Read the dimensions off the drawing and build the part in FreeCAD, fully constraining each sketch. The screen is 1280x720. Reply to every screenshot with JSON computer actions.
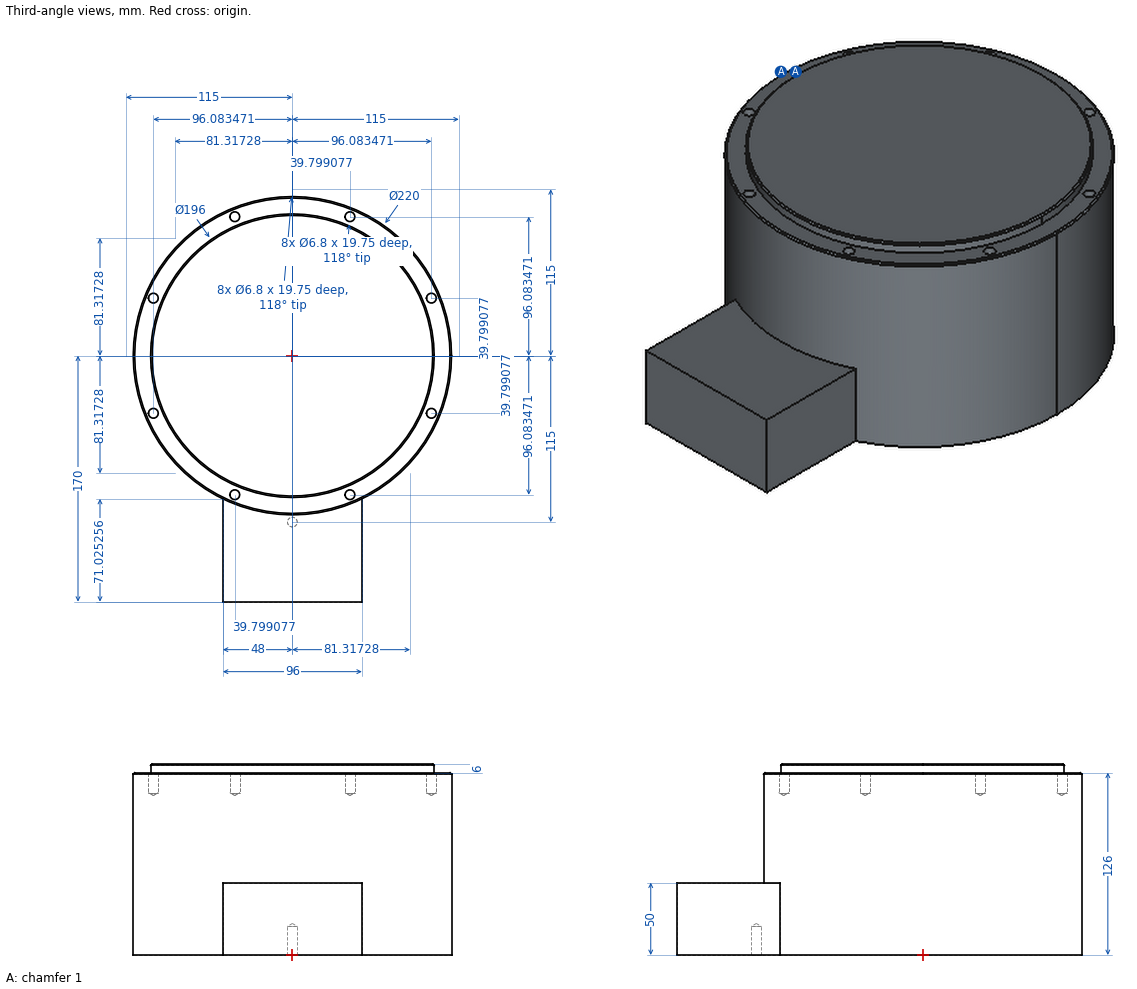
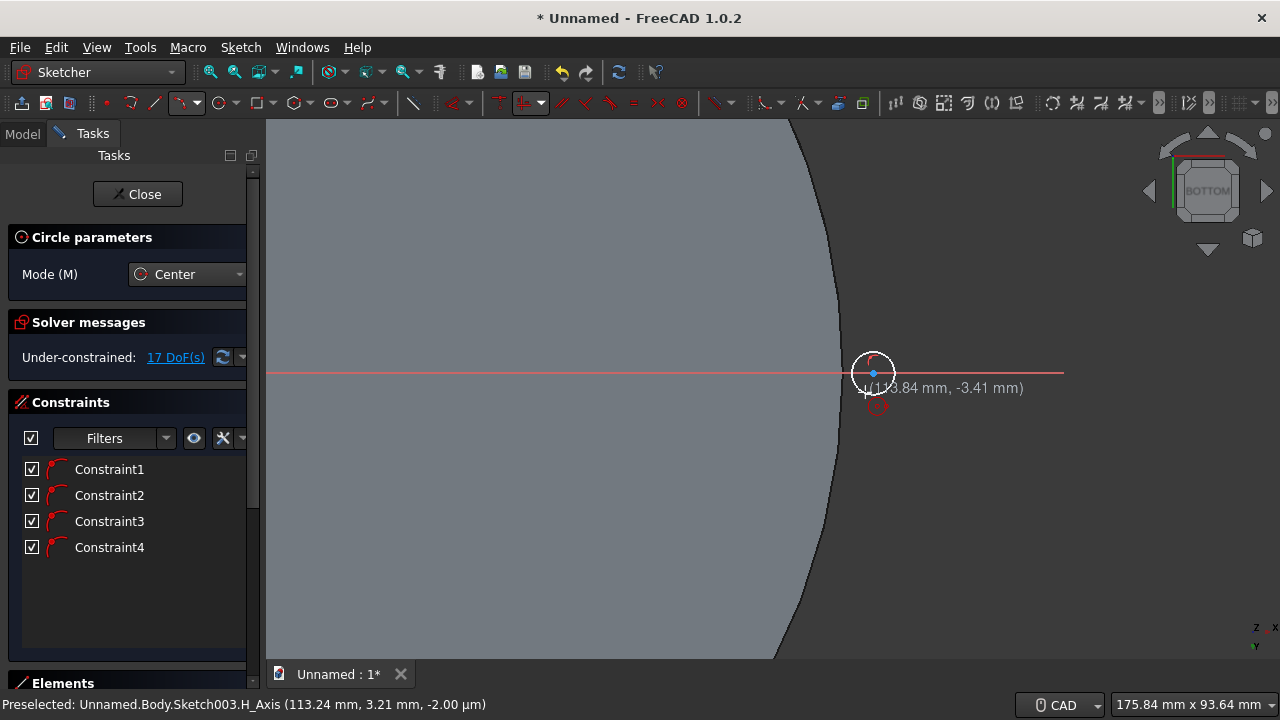
{"action": "scroll", "coordinate": [867, 394], "scroll_direction": "down", "scroll_amount": 7}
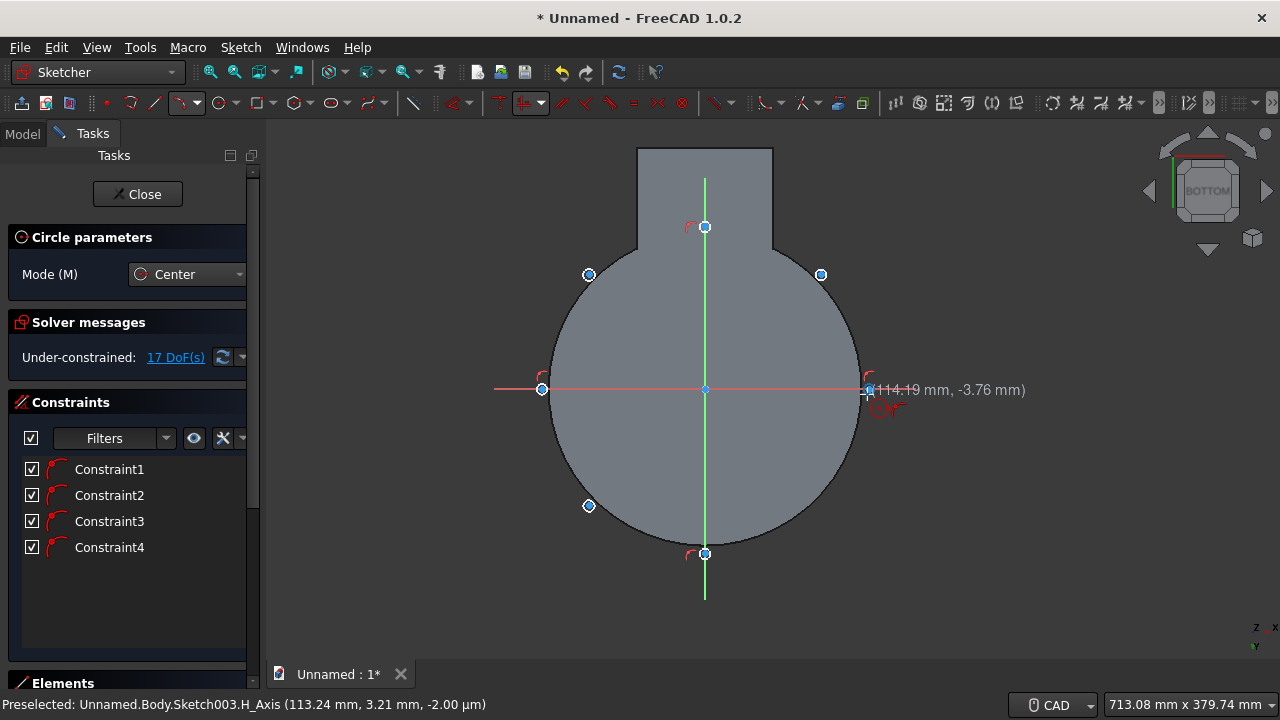
{"action": "scroll", "coordinate": [821, 505], "scroll_direction": "up", "scroll_amount": 8}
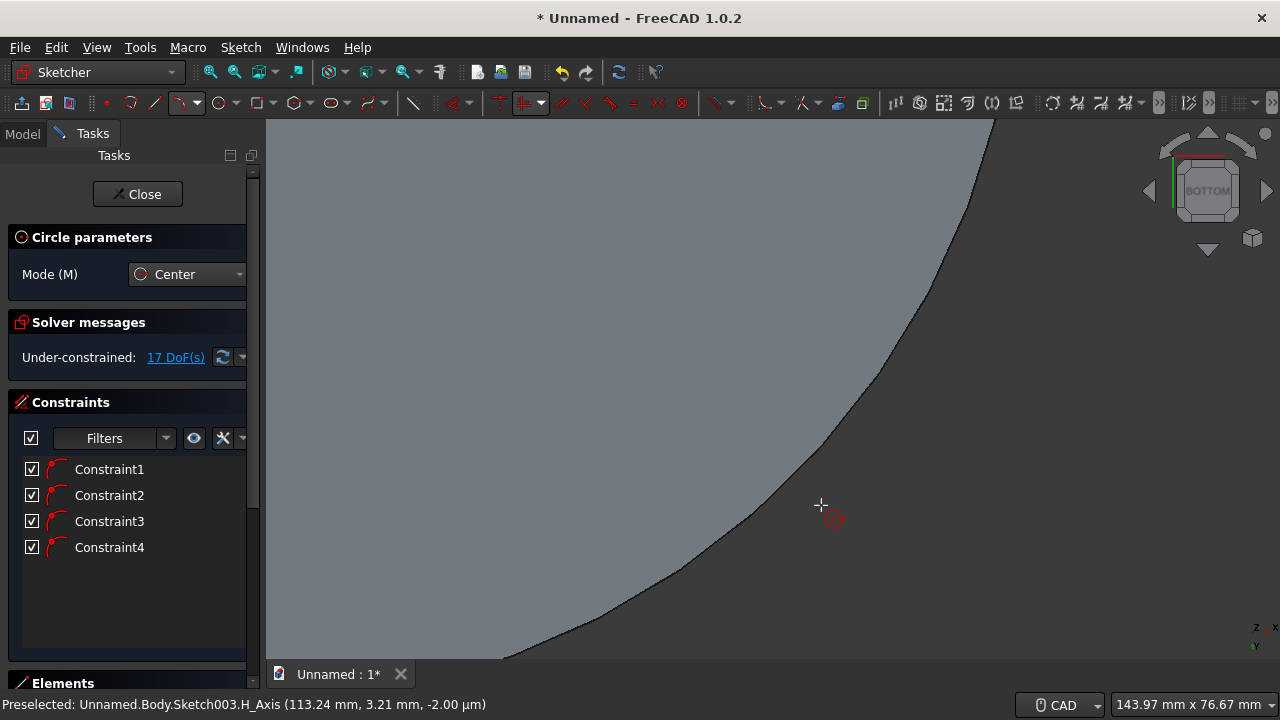
{"action": "scroll", "coordinate": [821, 505], "scroll_direction": "down", "scroll_amount": 8}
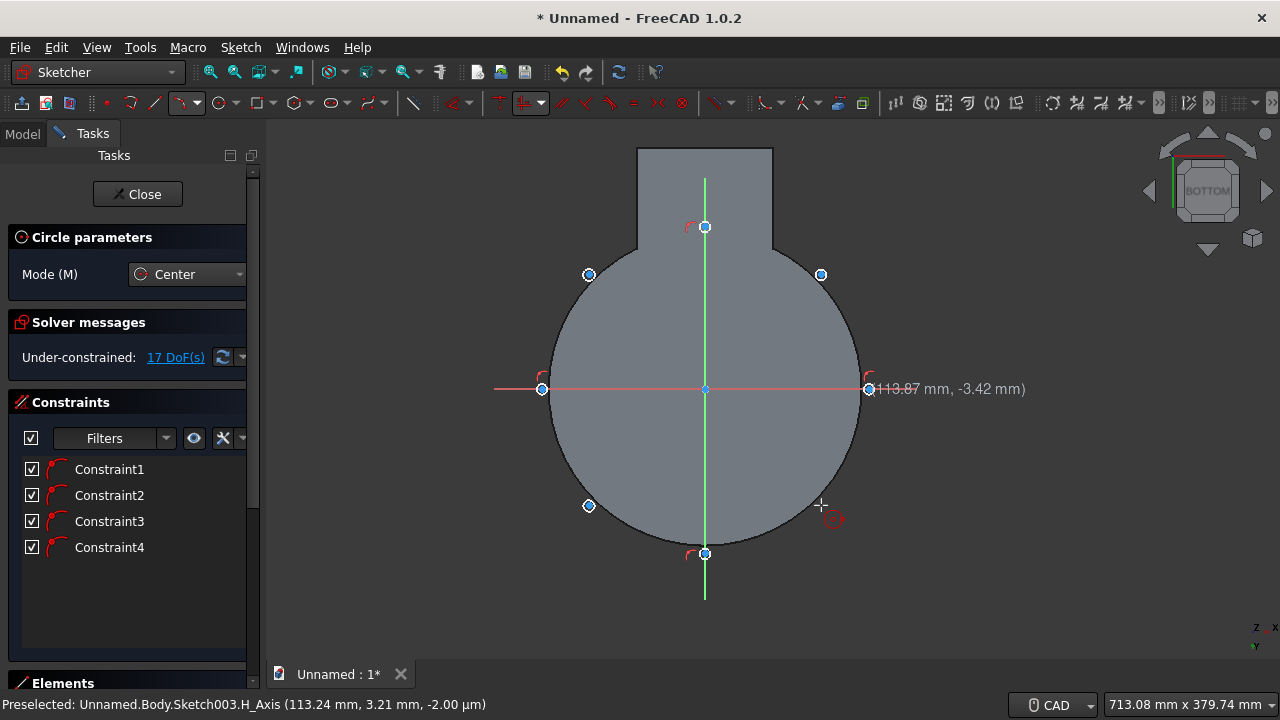
{"action": "left_click", "coordinate": [821, 505]}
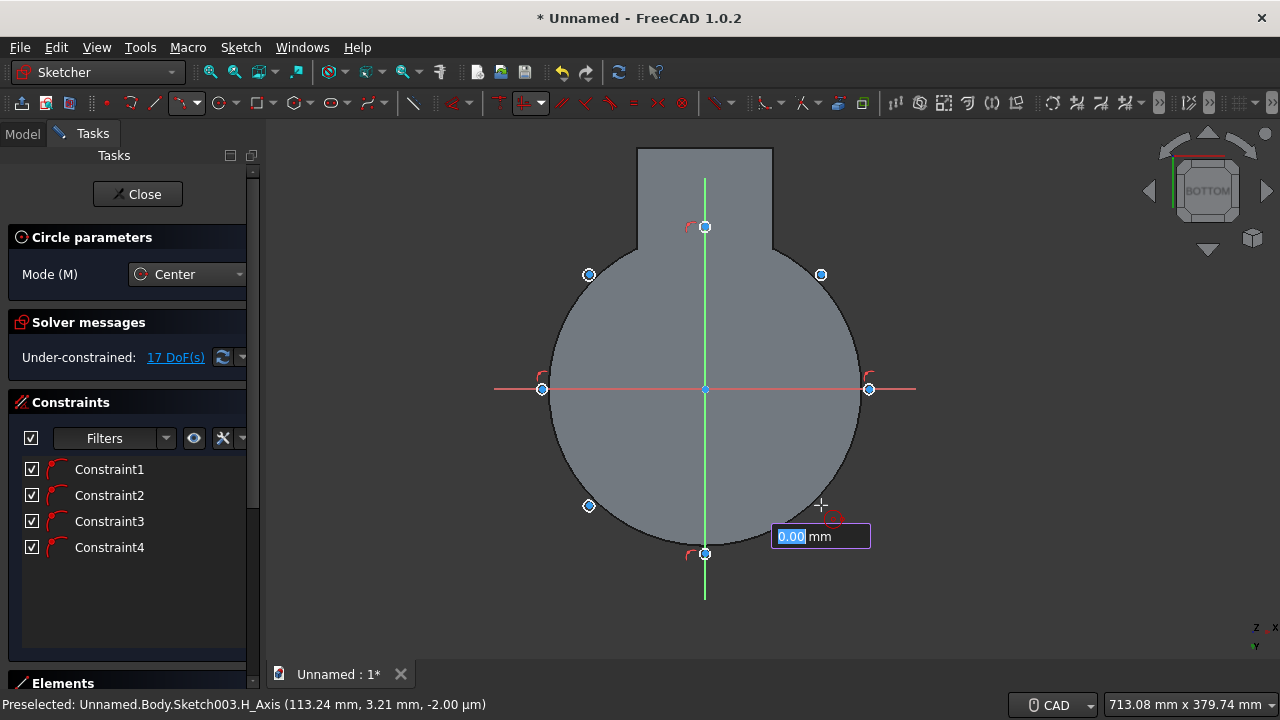
{"action": "scroll", "coordinate": [824, 502], "scroll_direction": "up", "scroll_amount": 6}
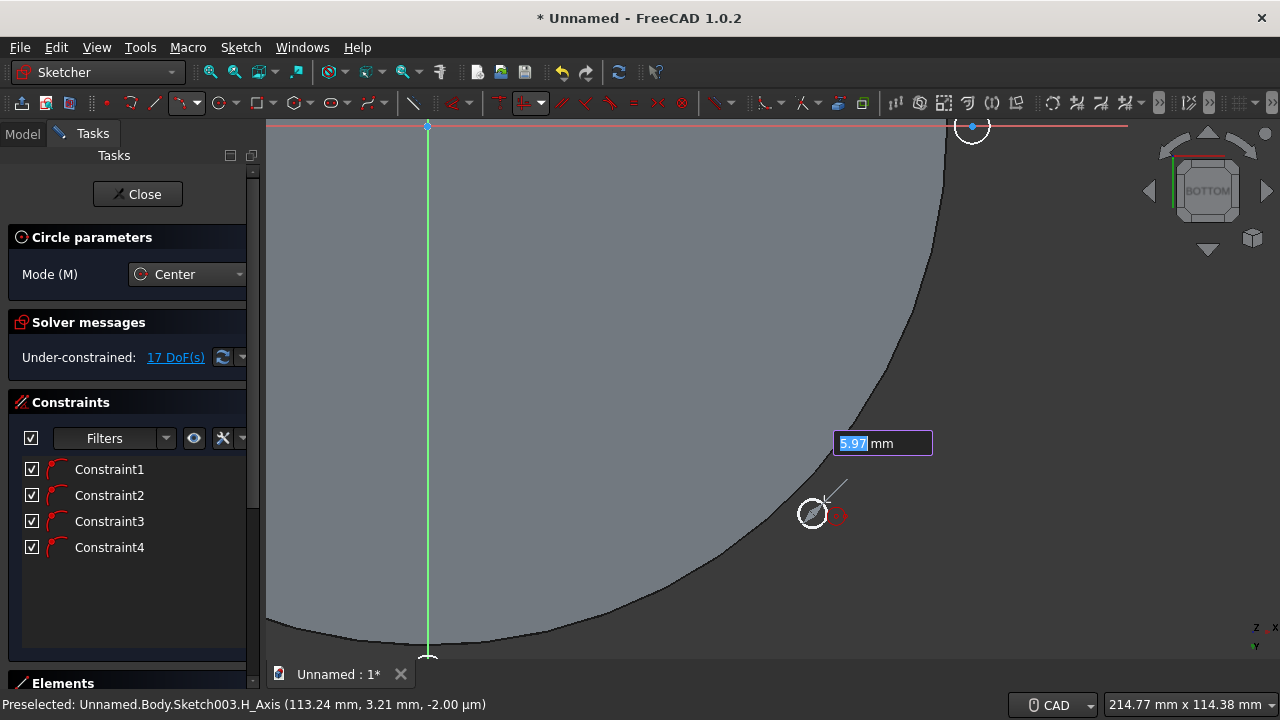
{"action": "left_click", "coordinate": [823, 499]}
{"action": "key", "text": "Escape"}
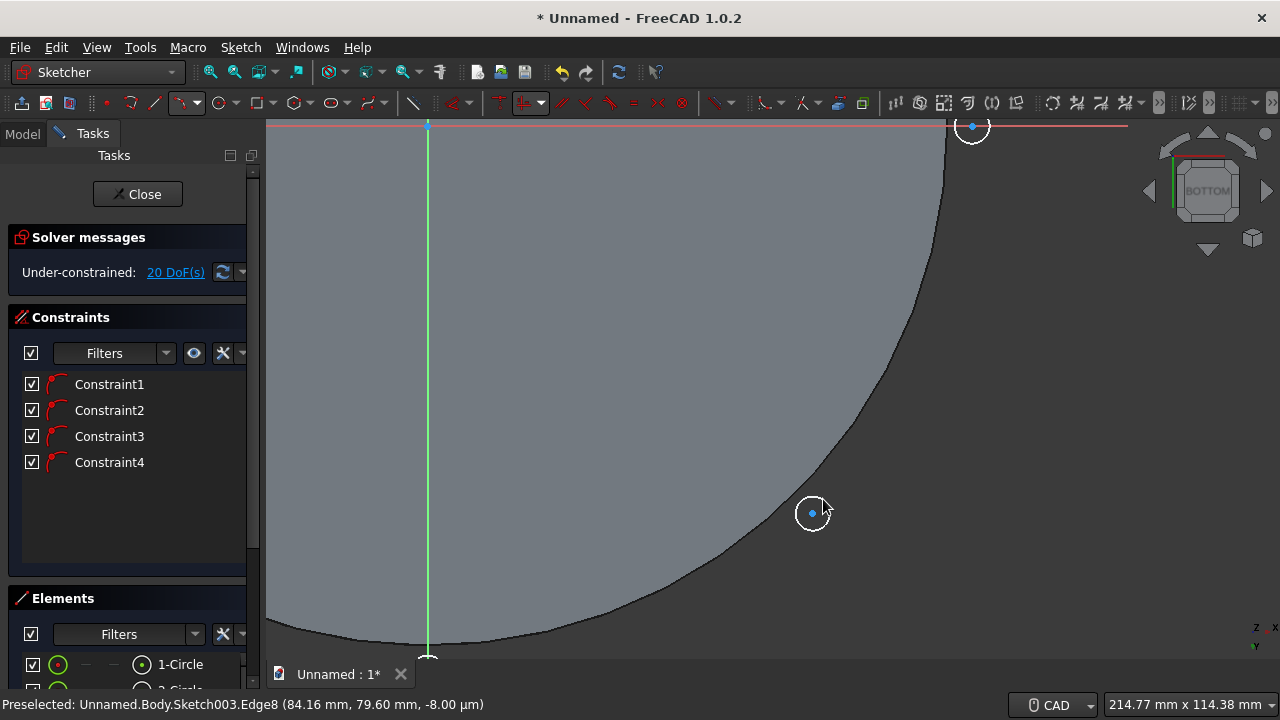
{"action": "scroll", "coordinate": [824, 502], "scroll_direction": "down", "scroll_amount": 6}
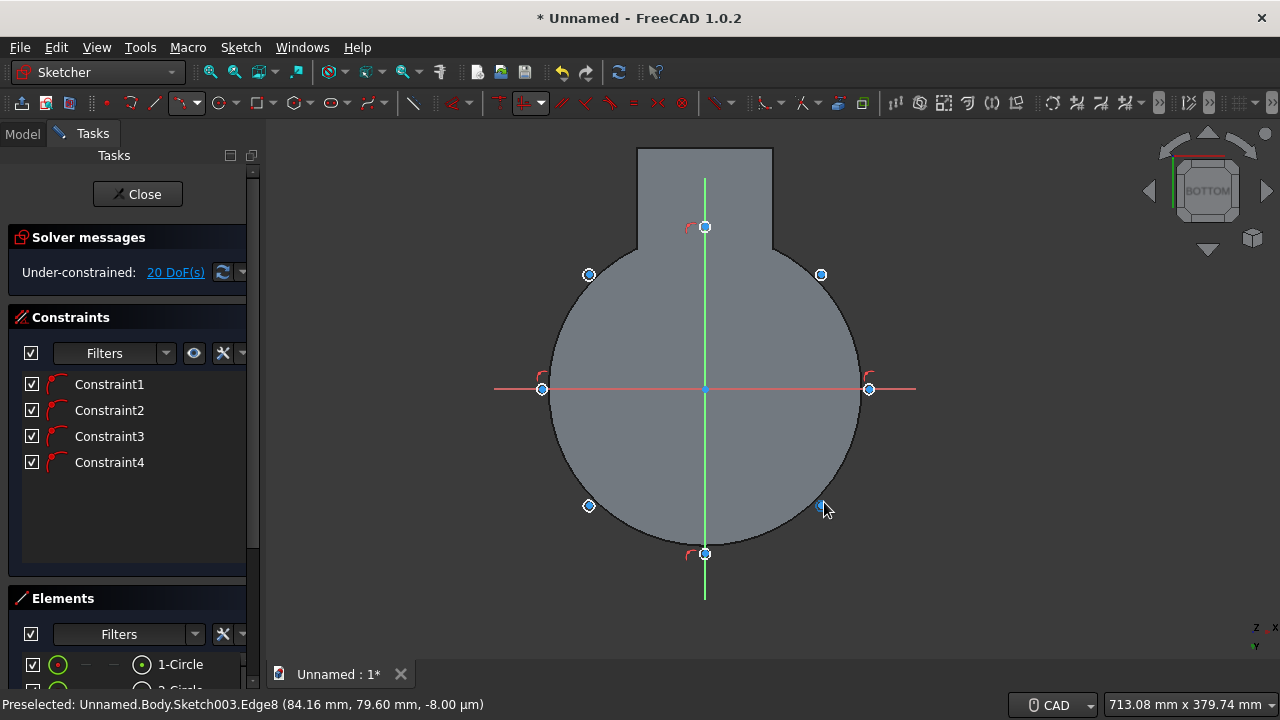
{"action": "scroll", "coordinate": [709, 550], "scroll_direction": "up", "scroll_amount": 7}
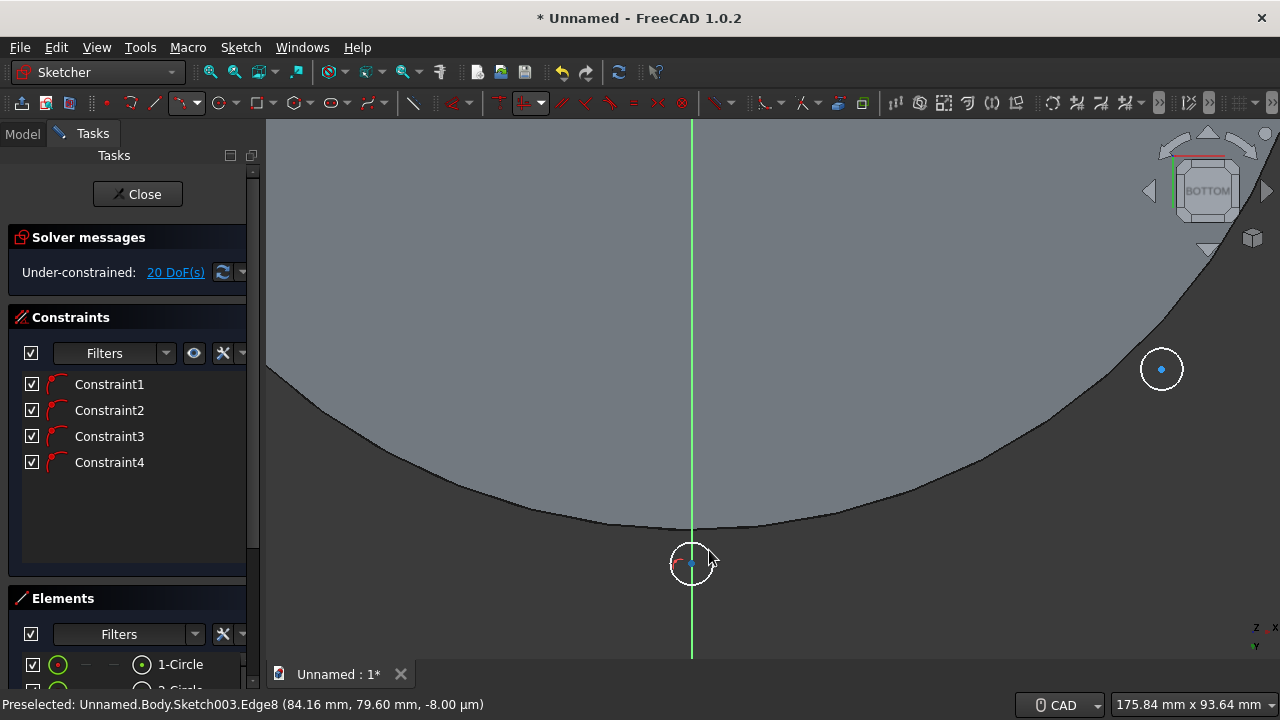
{"action": "left_click", "coordinate": [707, 549]}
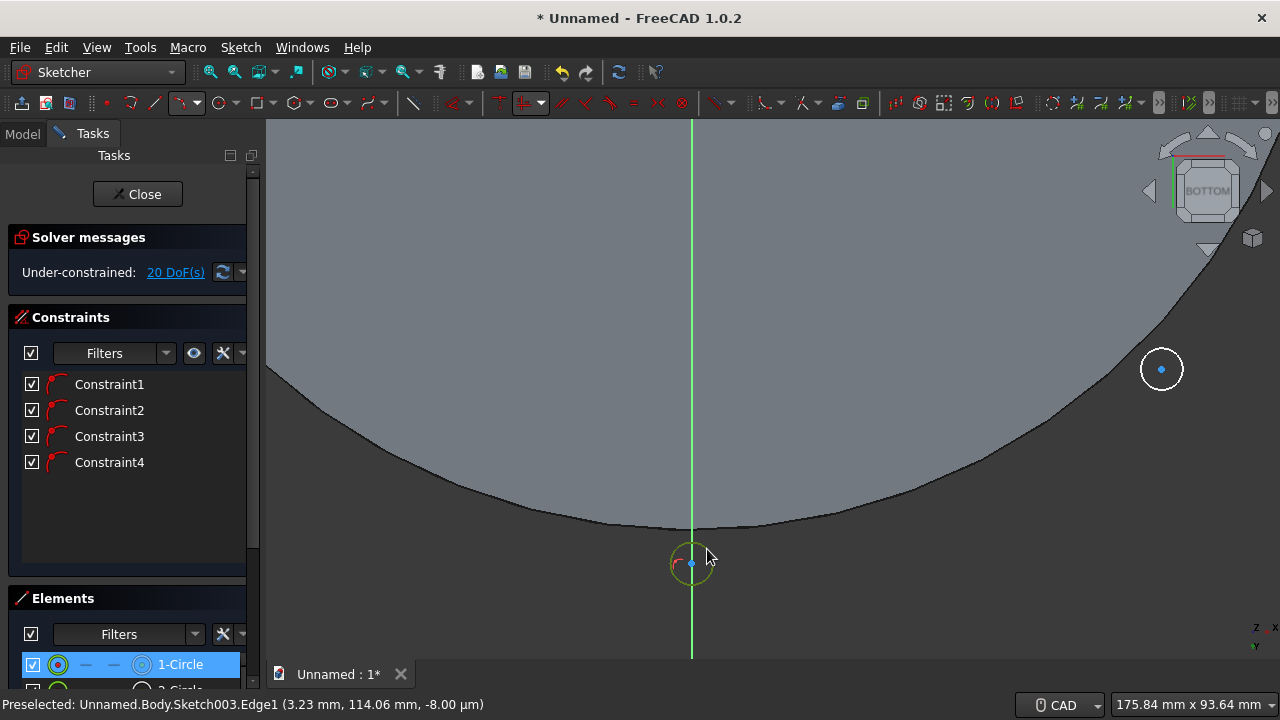
{"action": "scroll", "coordinate": [709, 550], "scroll_direction": "down", "scroll_amount": 7}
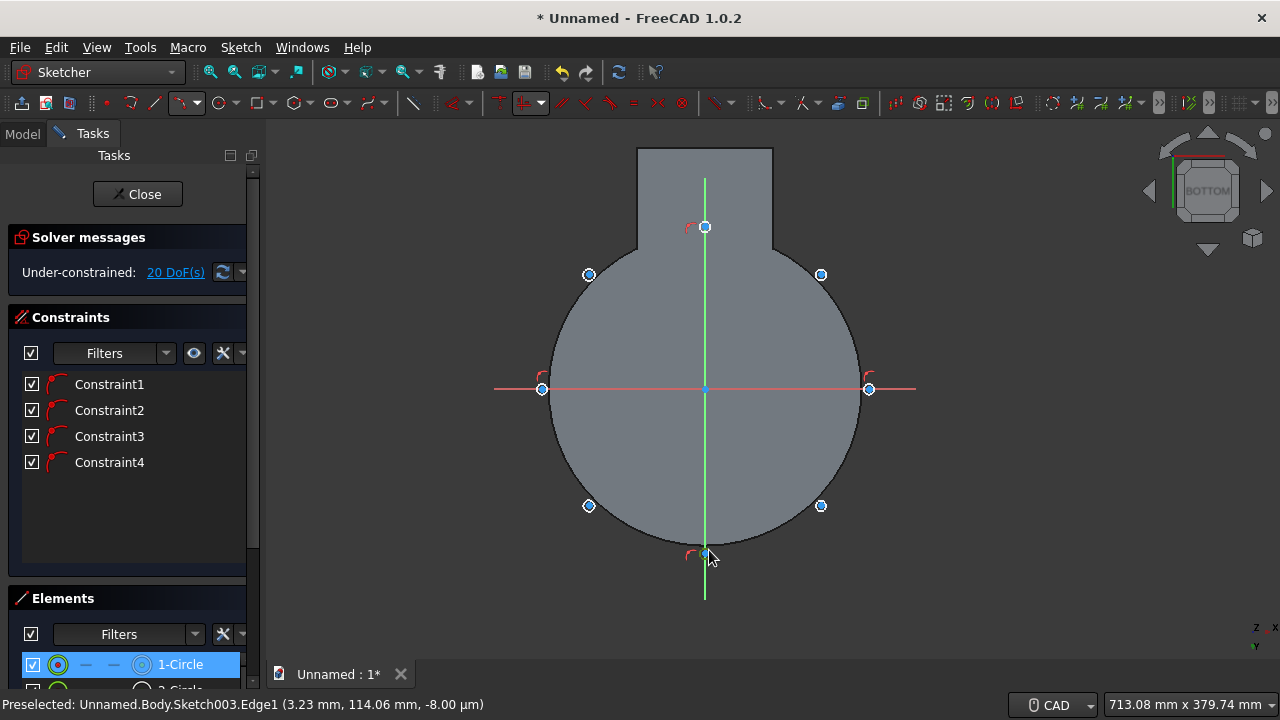
{"action": "scroll", "coordinate": [593, 502], "scroll_direction": "up", "scroll_amount": 5}